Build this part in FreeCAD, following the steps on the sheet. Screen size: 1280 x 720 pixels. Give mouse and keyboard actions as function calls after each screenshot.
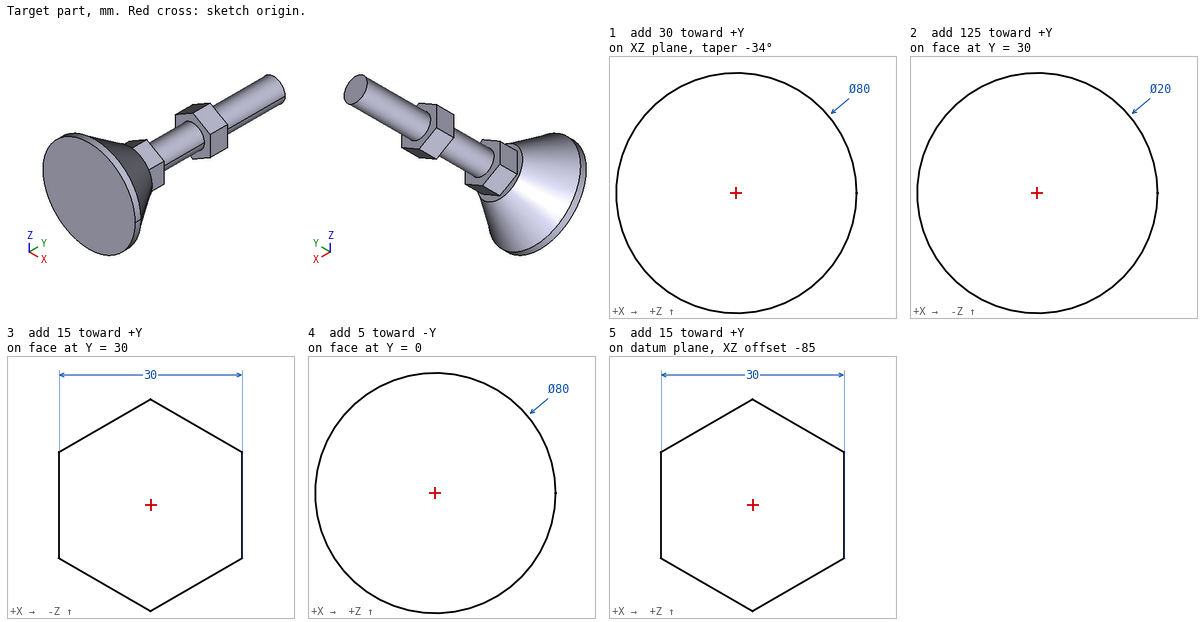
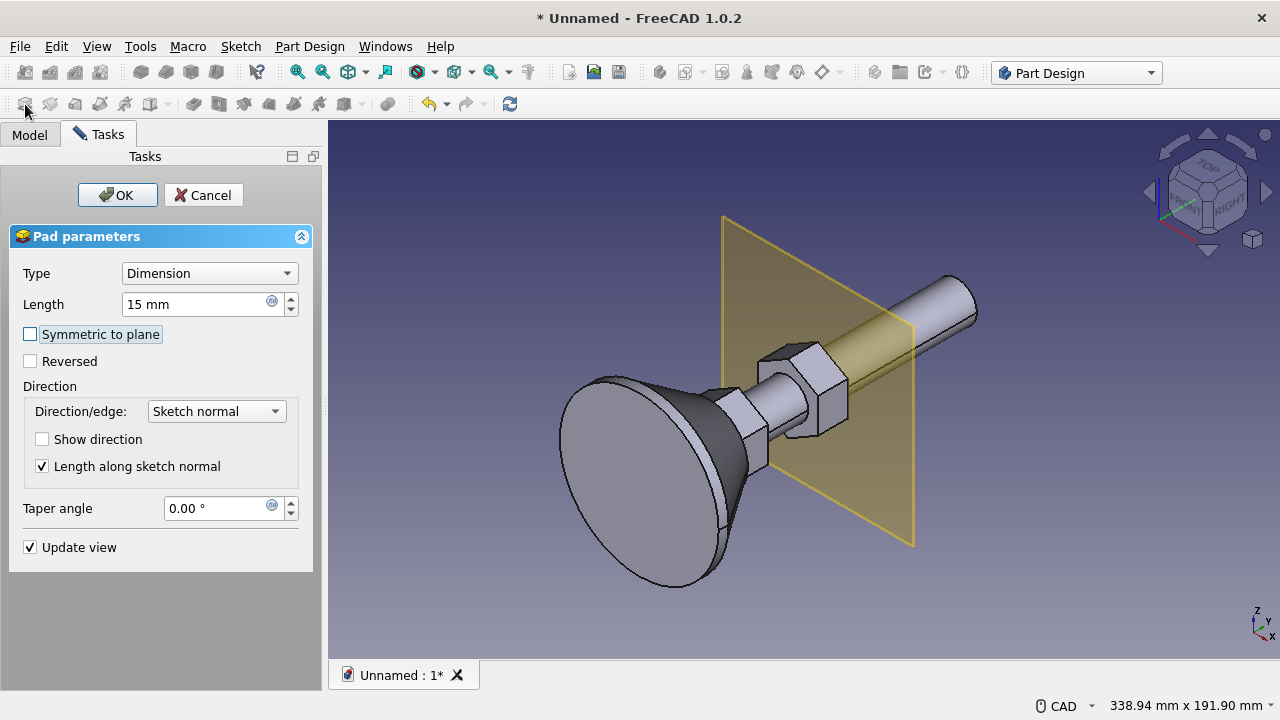
click(31, 361)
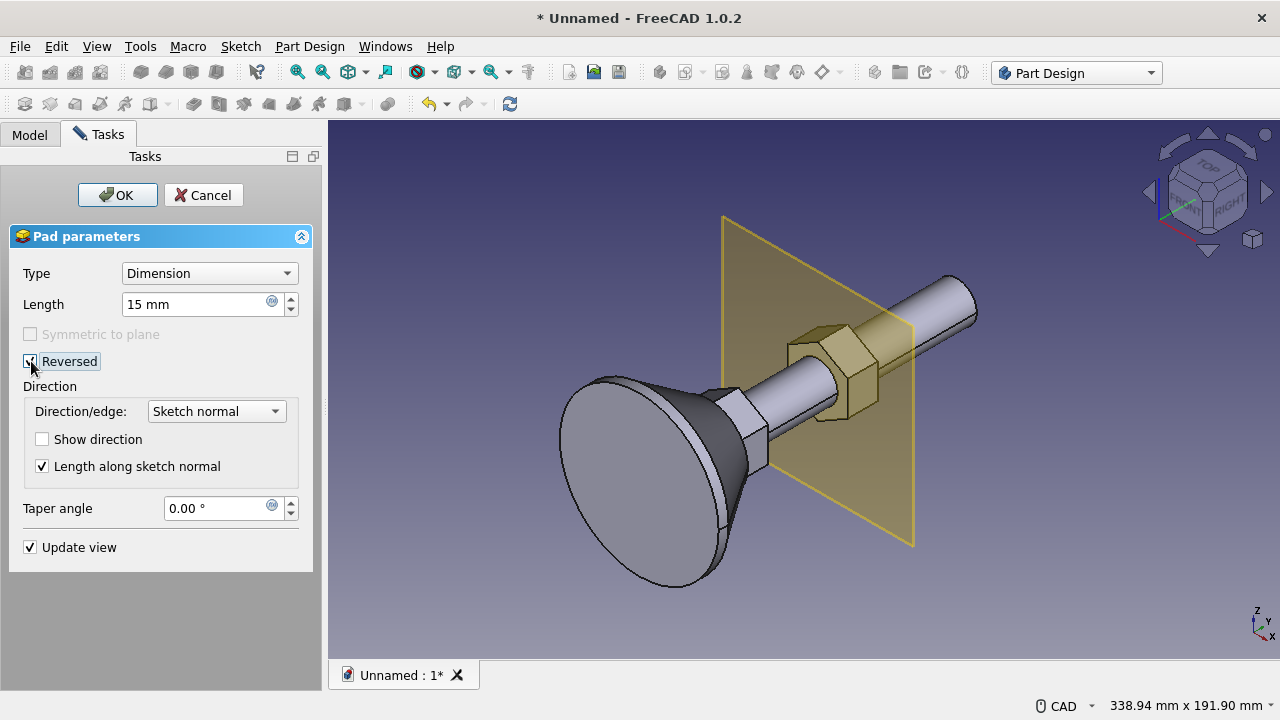
click(118, 195)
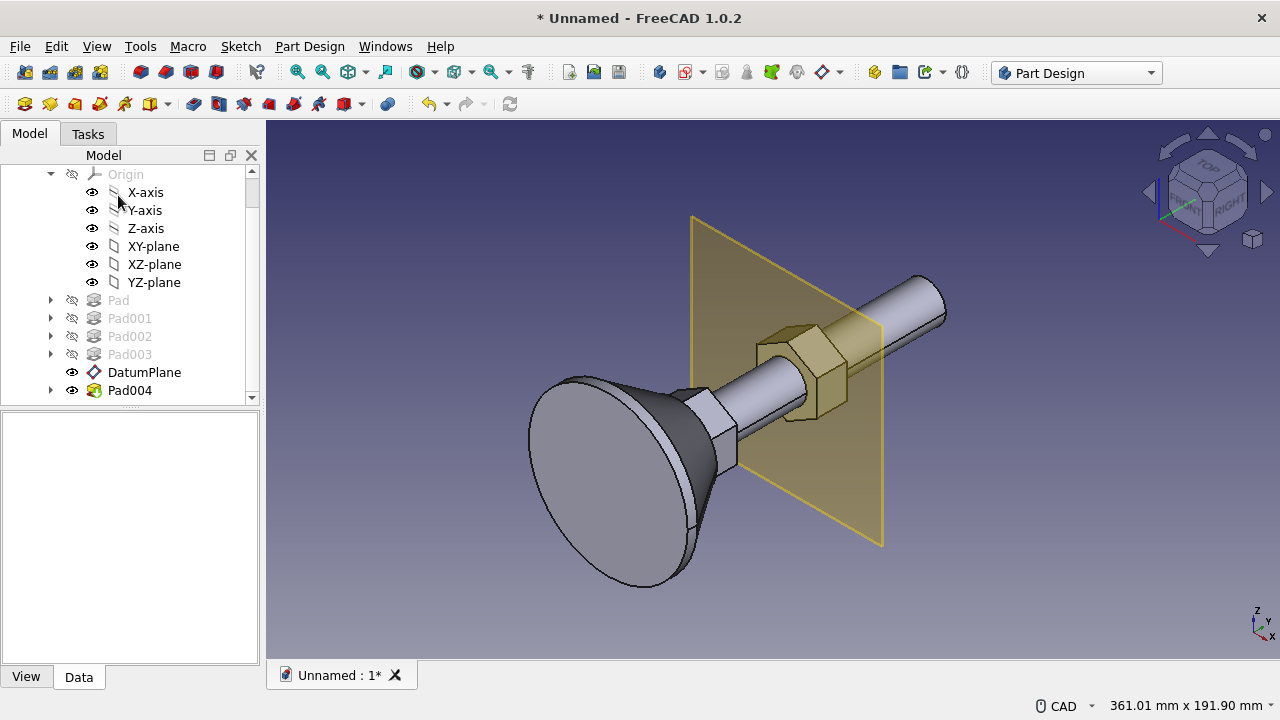
click(117, 372)
key(space)